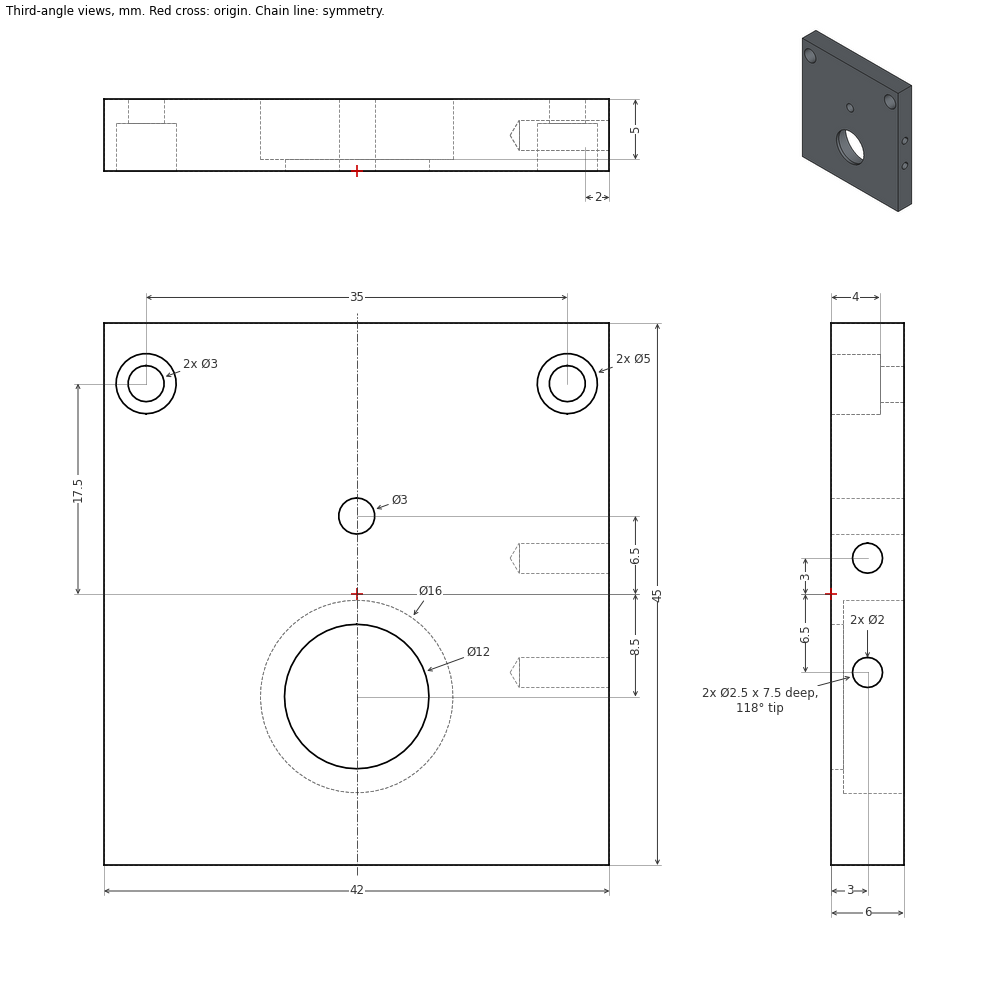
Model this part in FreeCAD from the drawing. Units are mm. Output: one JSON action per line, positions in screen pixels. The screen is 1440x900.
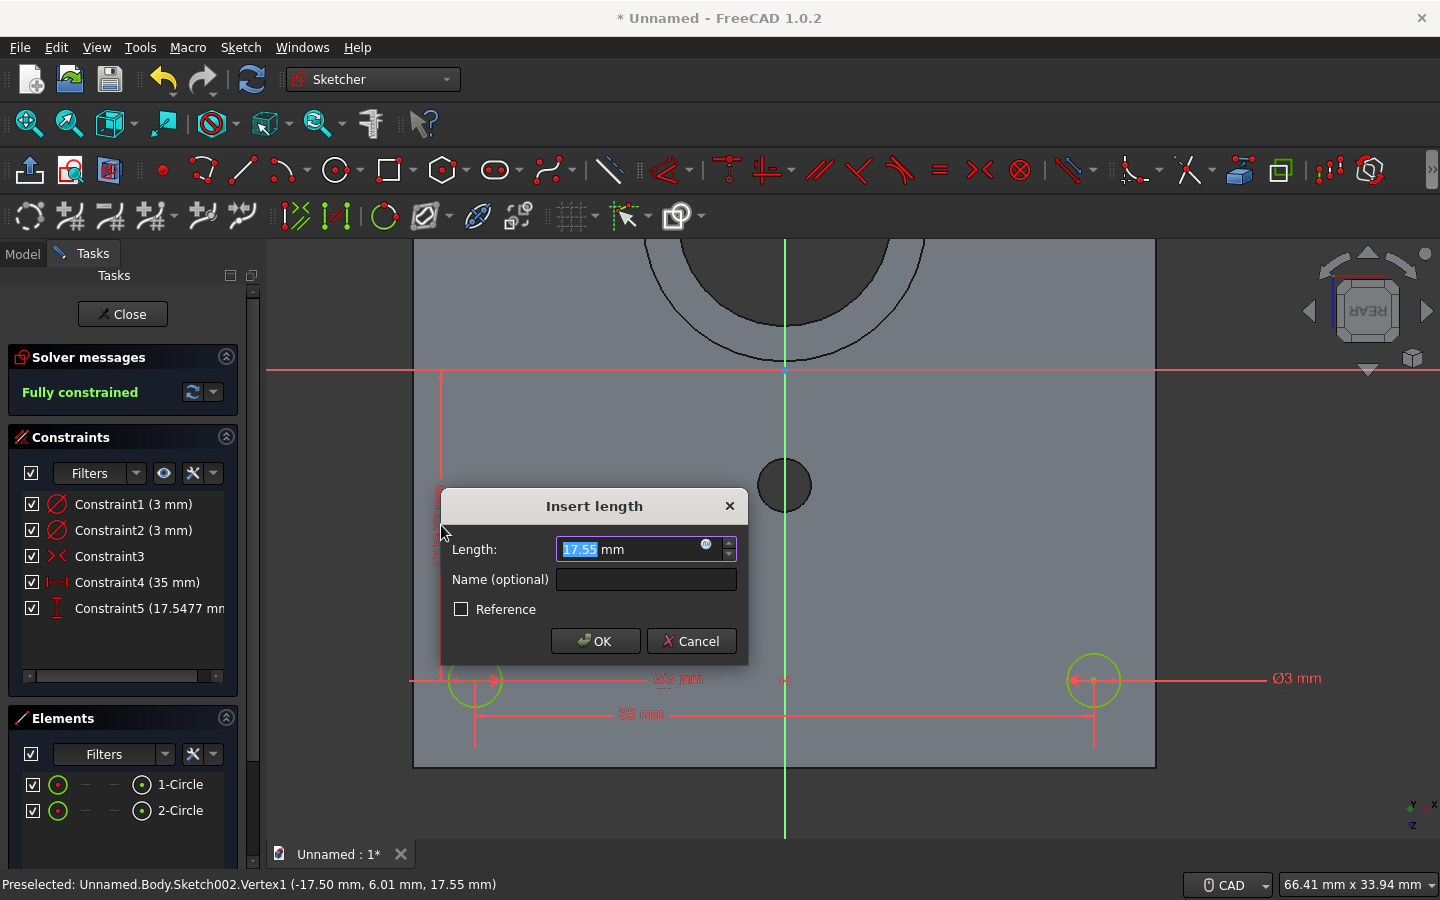
{"action": "type", "text": "17.5"}
{"action": "key", "text": "Return"}
{"action": "key", "text": "Escape"}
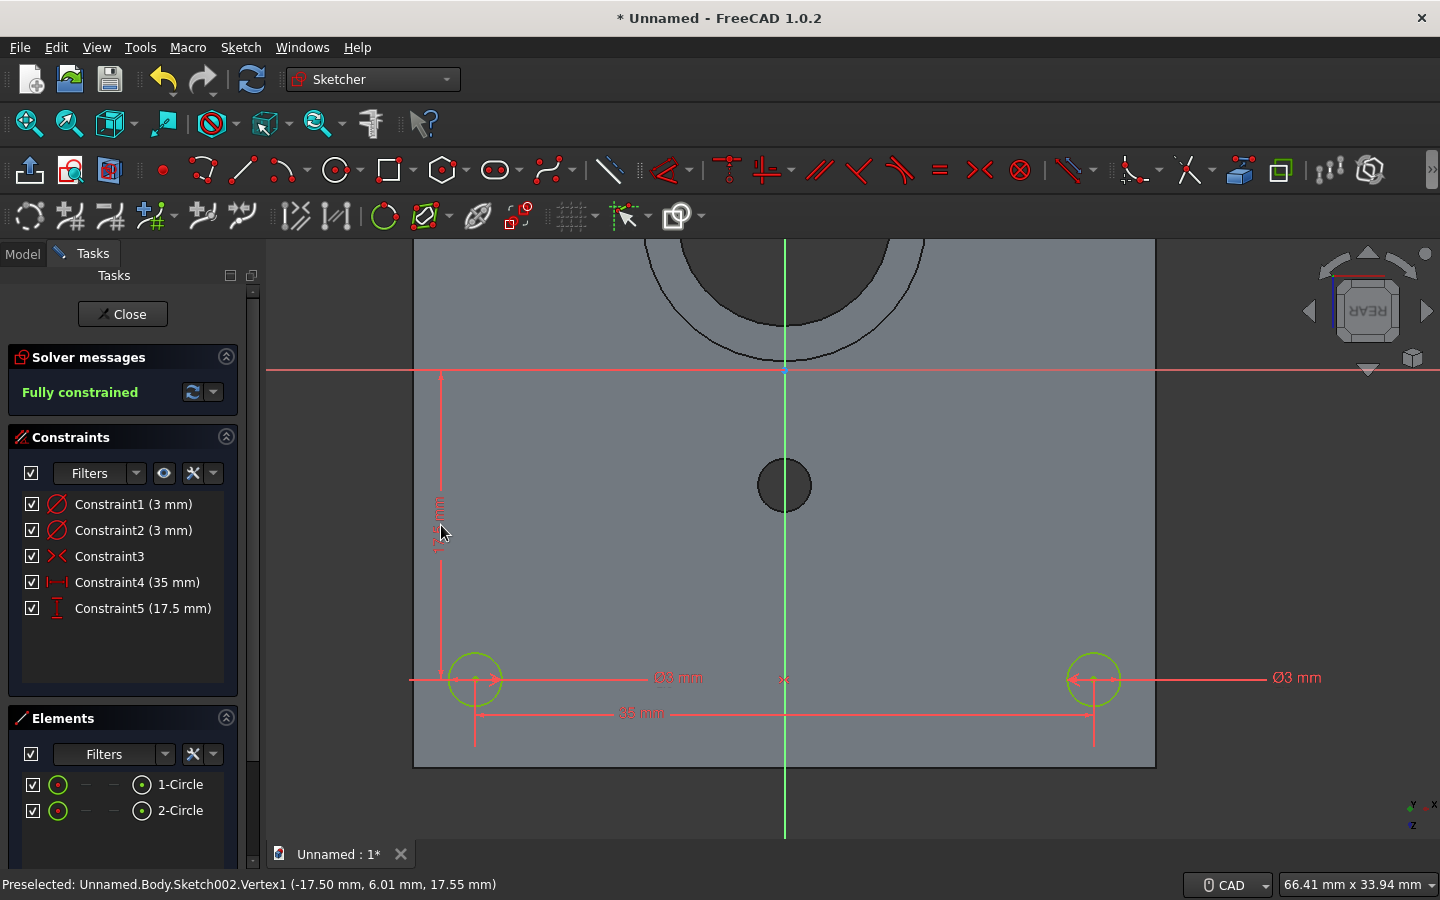
{"action": "left_click", "coordinate": [123, 314]}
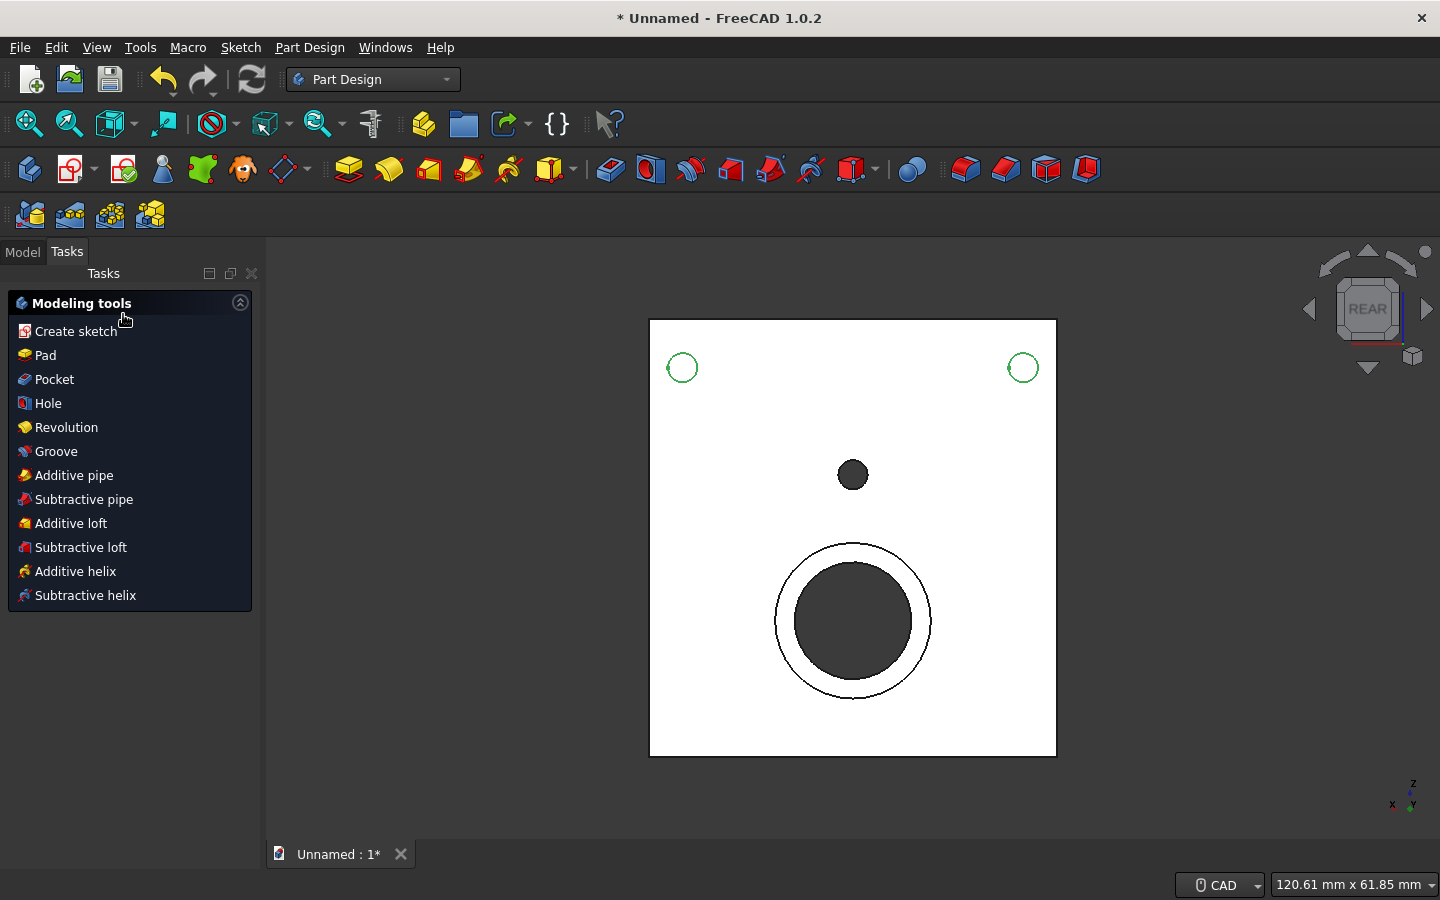
{"action": "left_click", "coordinate": [612, 170]}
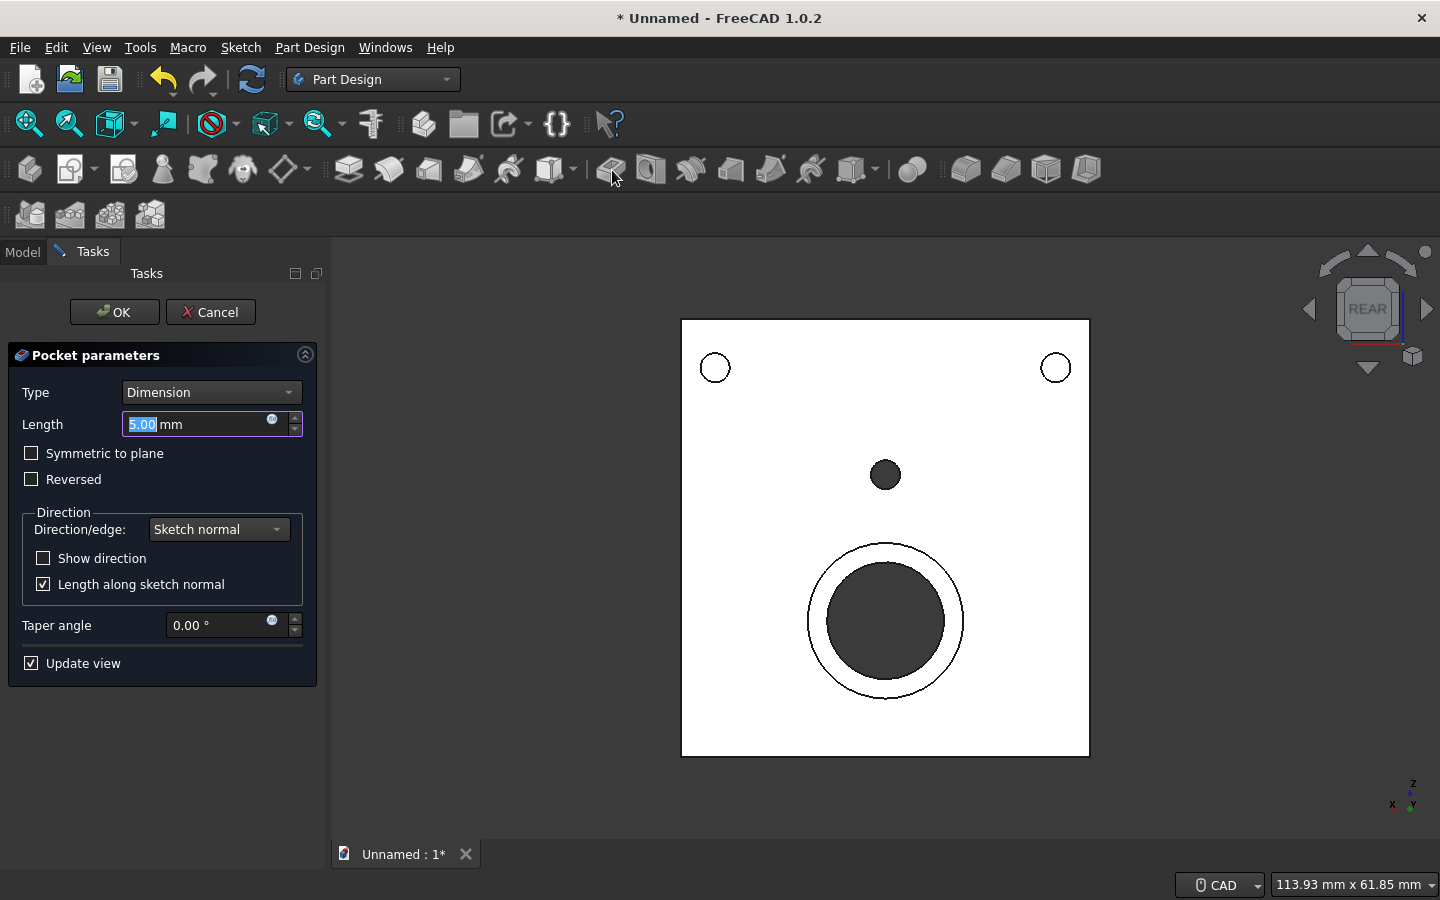
{"action": "left_click", "coordinate": [212, 392]}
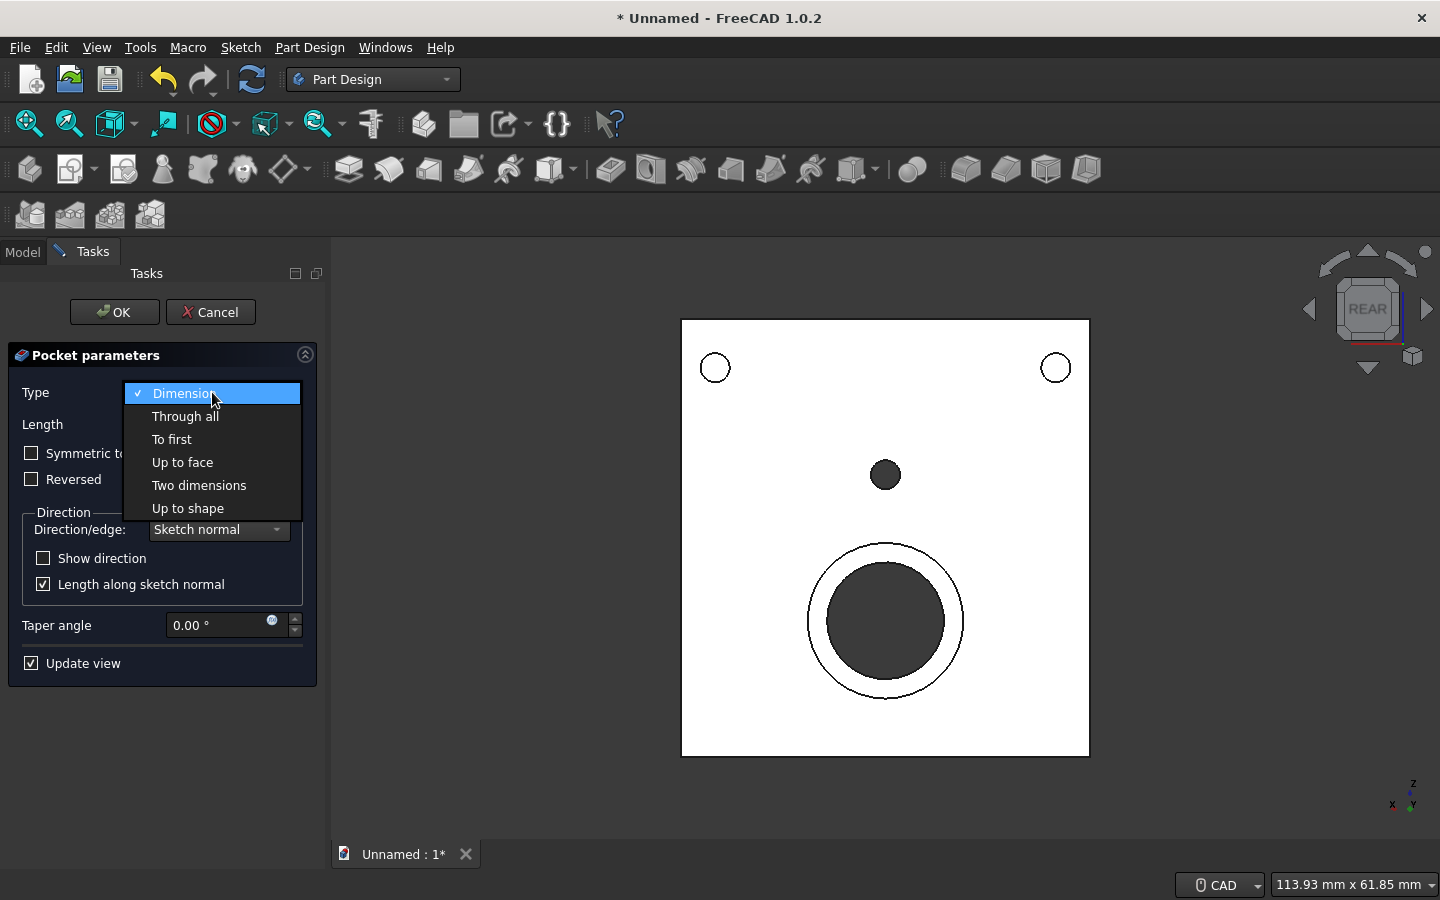
{"action": "left_click", "coordinate": [212, 416]}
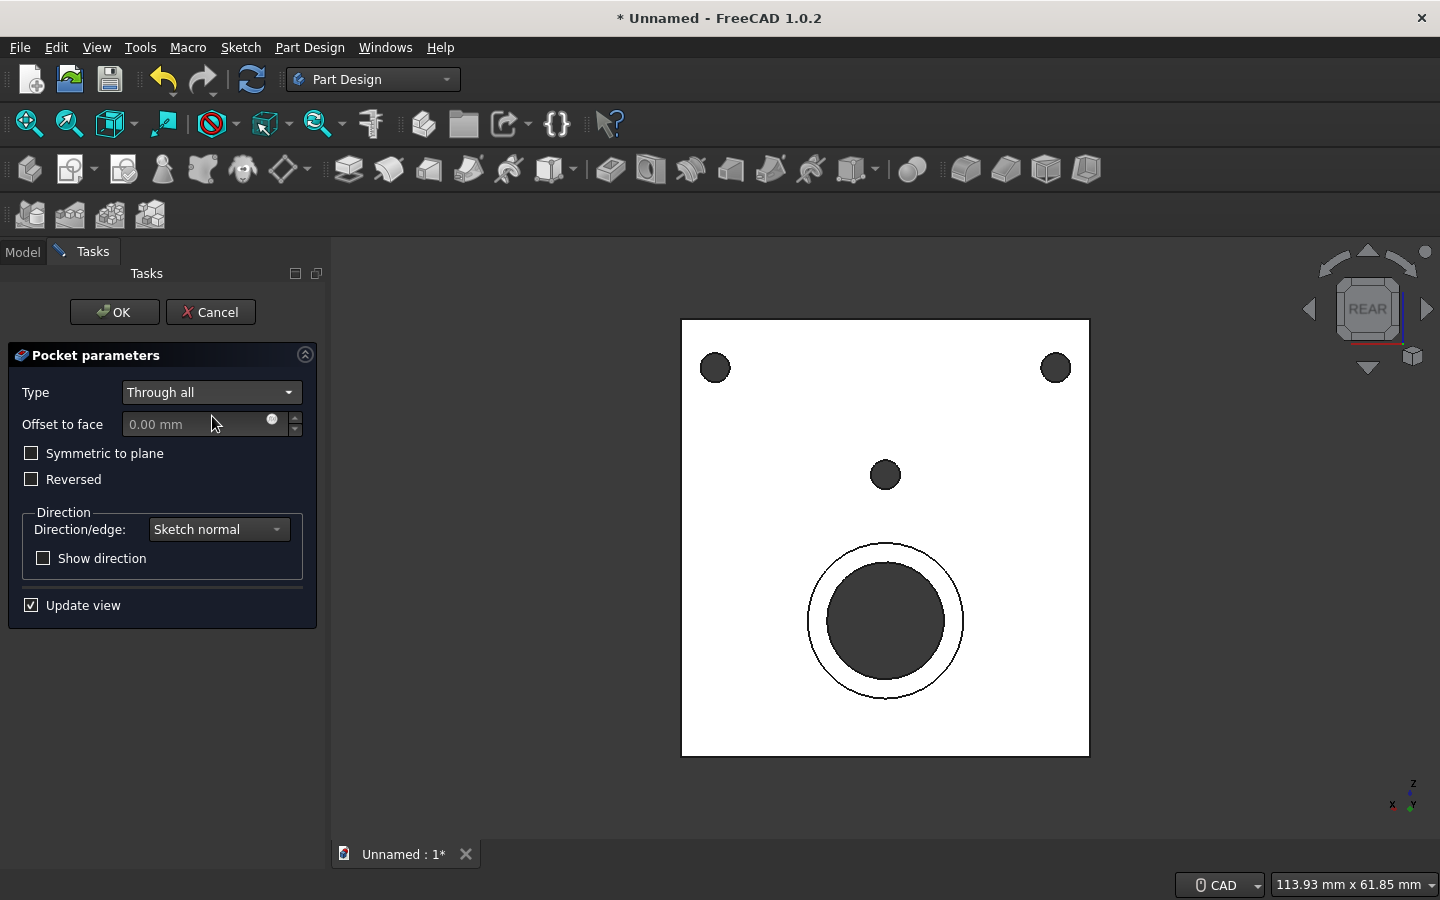
{"action": "left_click", "coordinate": [115, 312]}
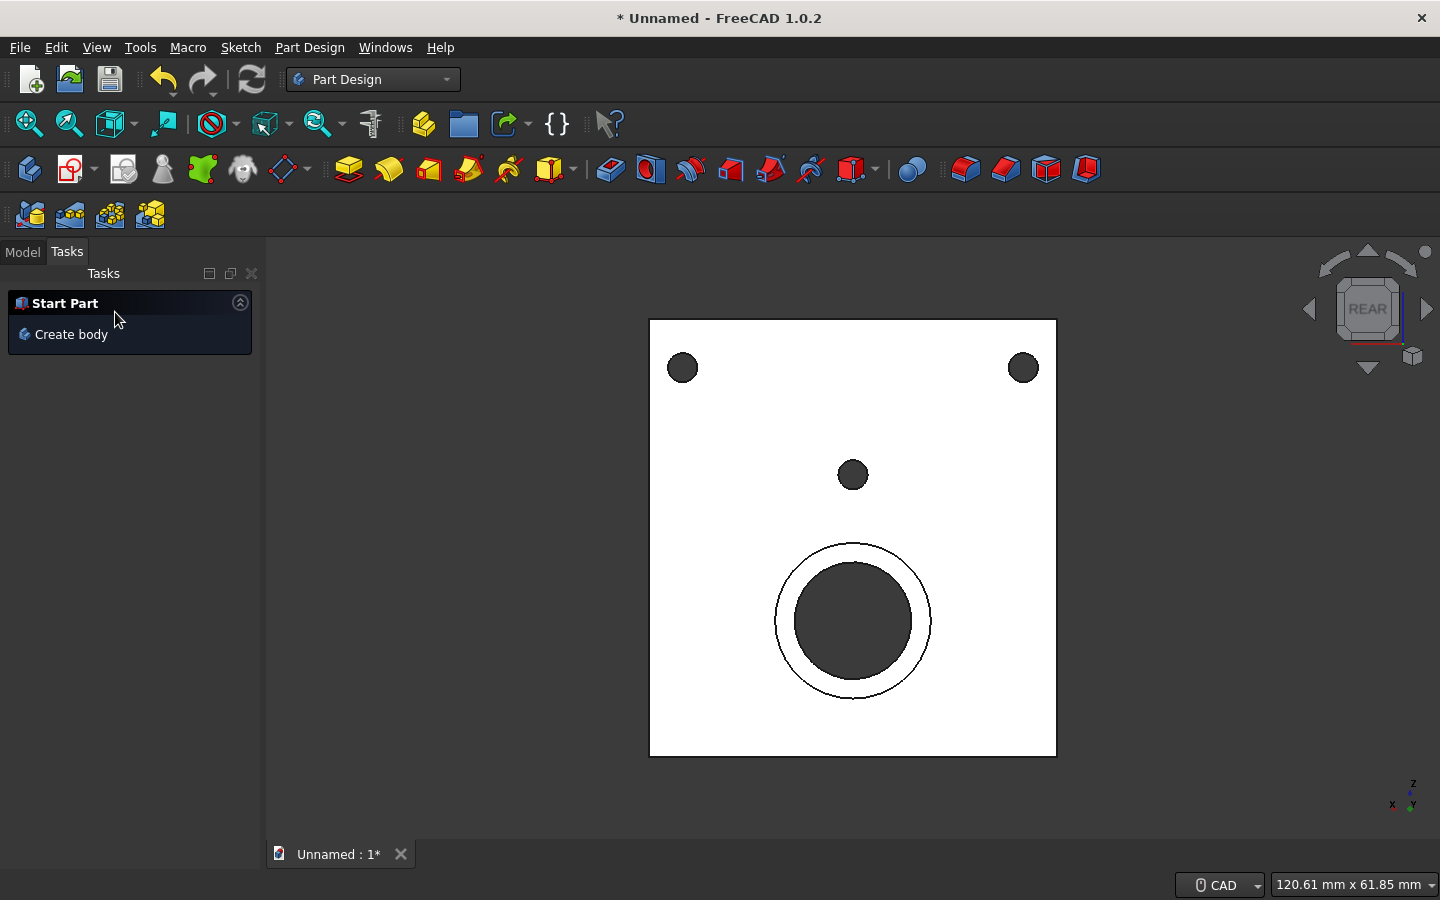
{"action": "left_click", "coordinate": [70, 170]}